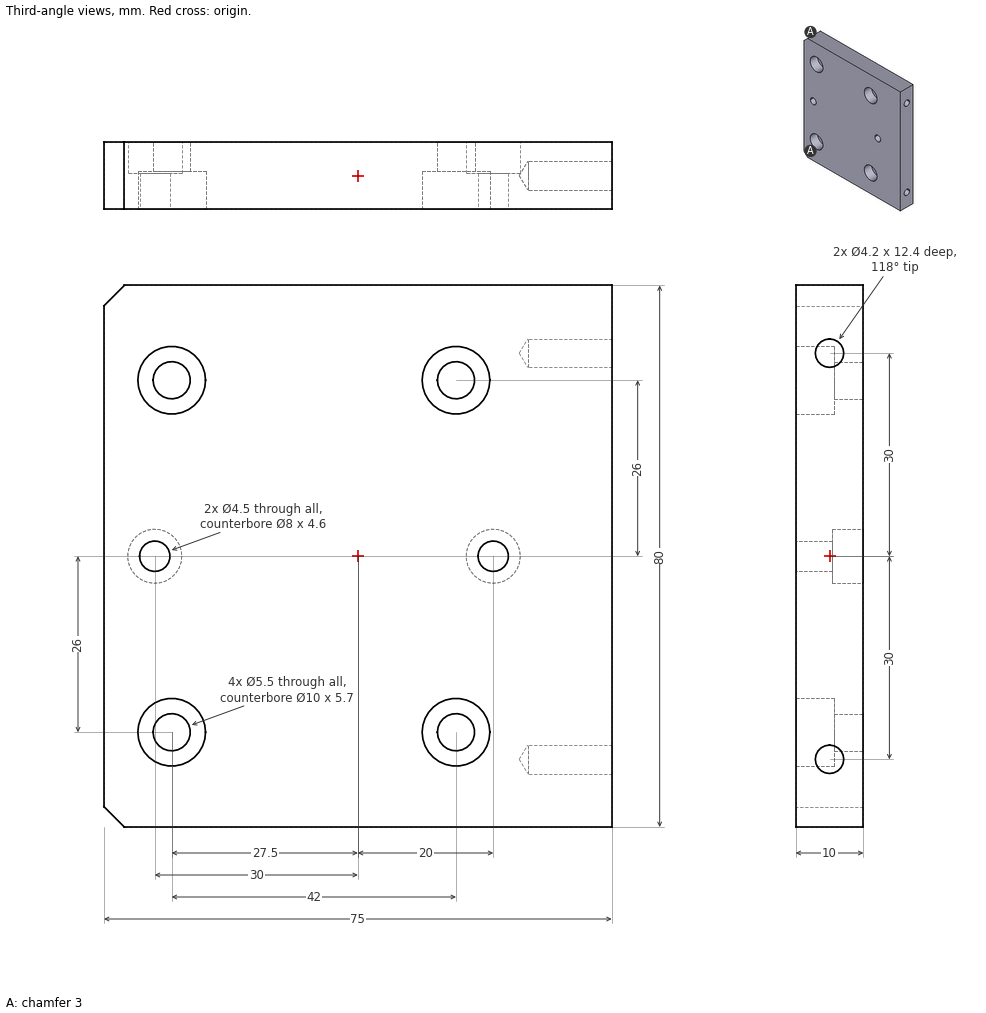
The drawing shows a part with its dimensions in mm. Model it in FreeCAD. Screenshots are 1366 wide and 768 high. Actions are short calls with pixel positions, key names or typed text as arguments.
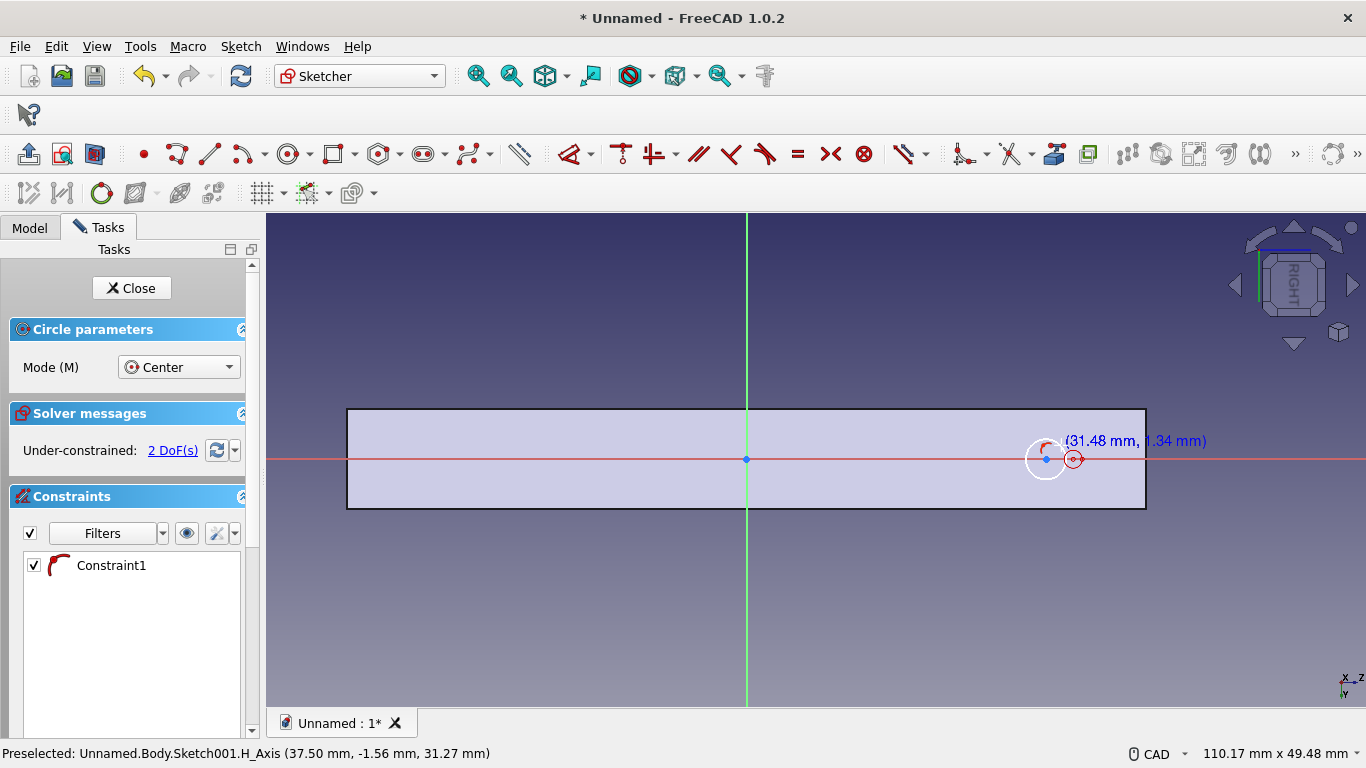
click(447, 459)
click(462, 445)
key(Escape)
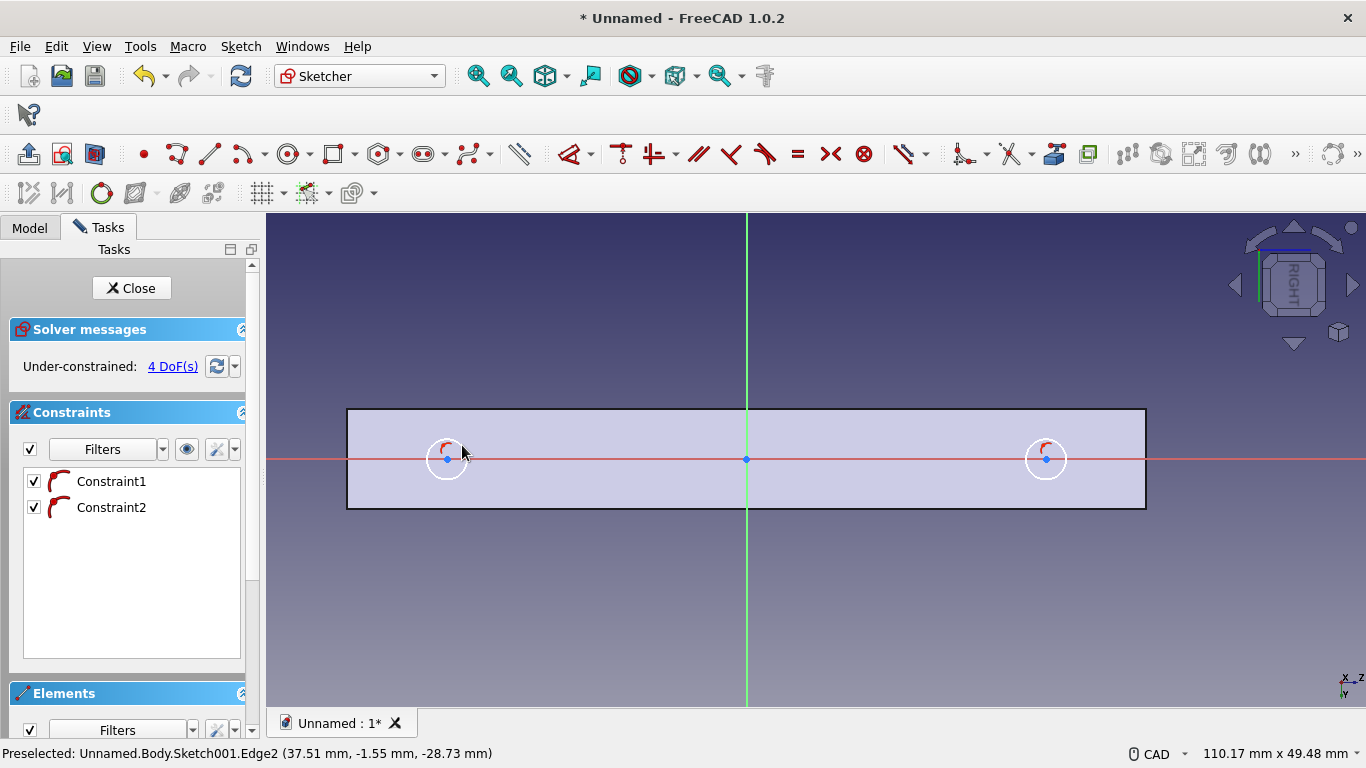
click(1060, 445)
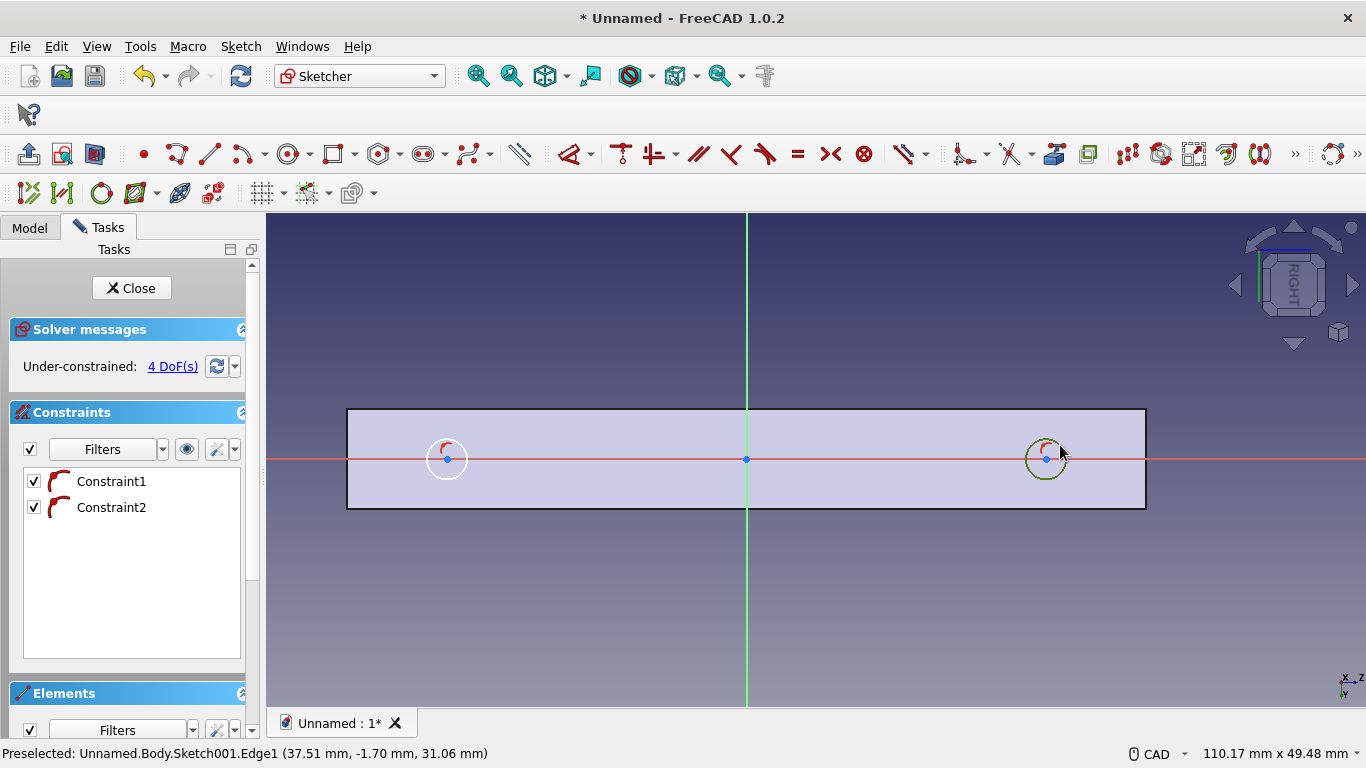
click(461, 445)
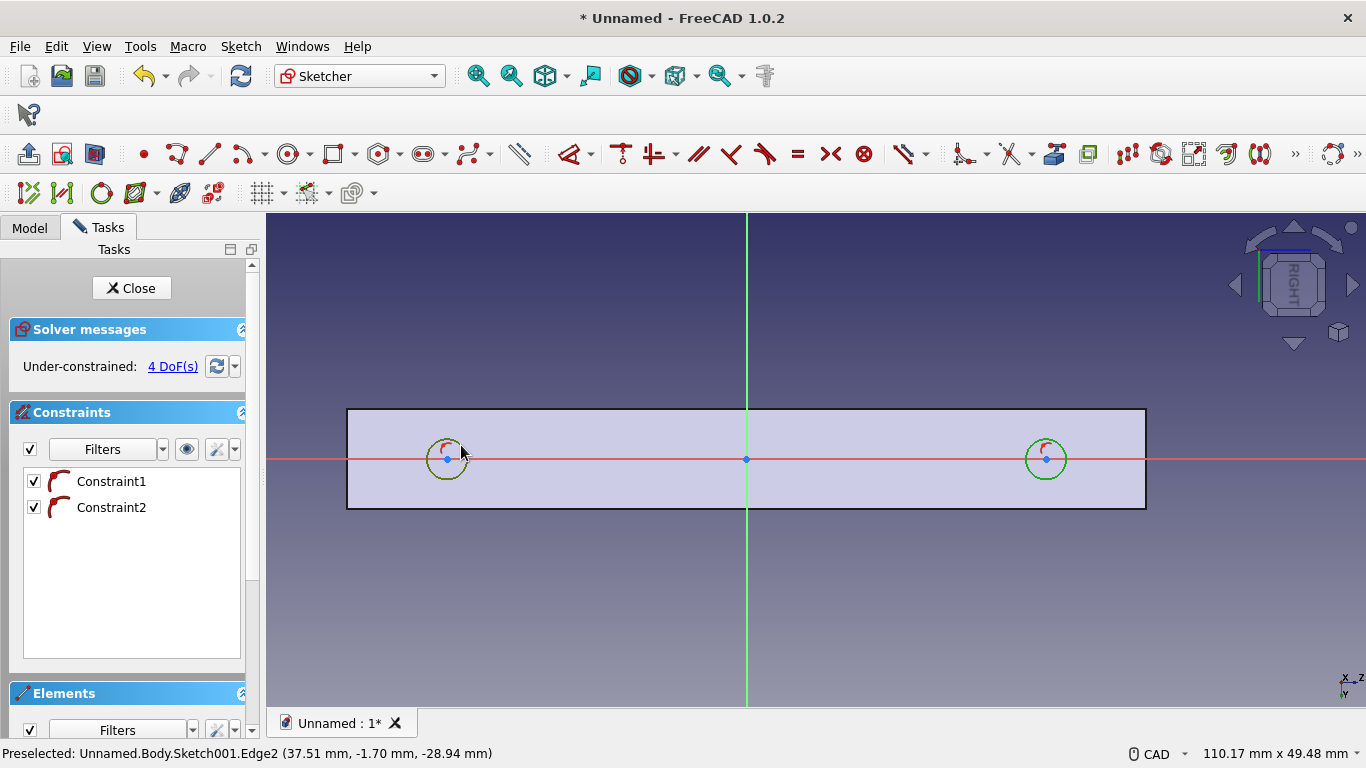
click(798, 154)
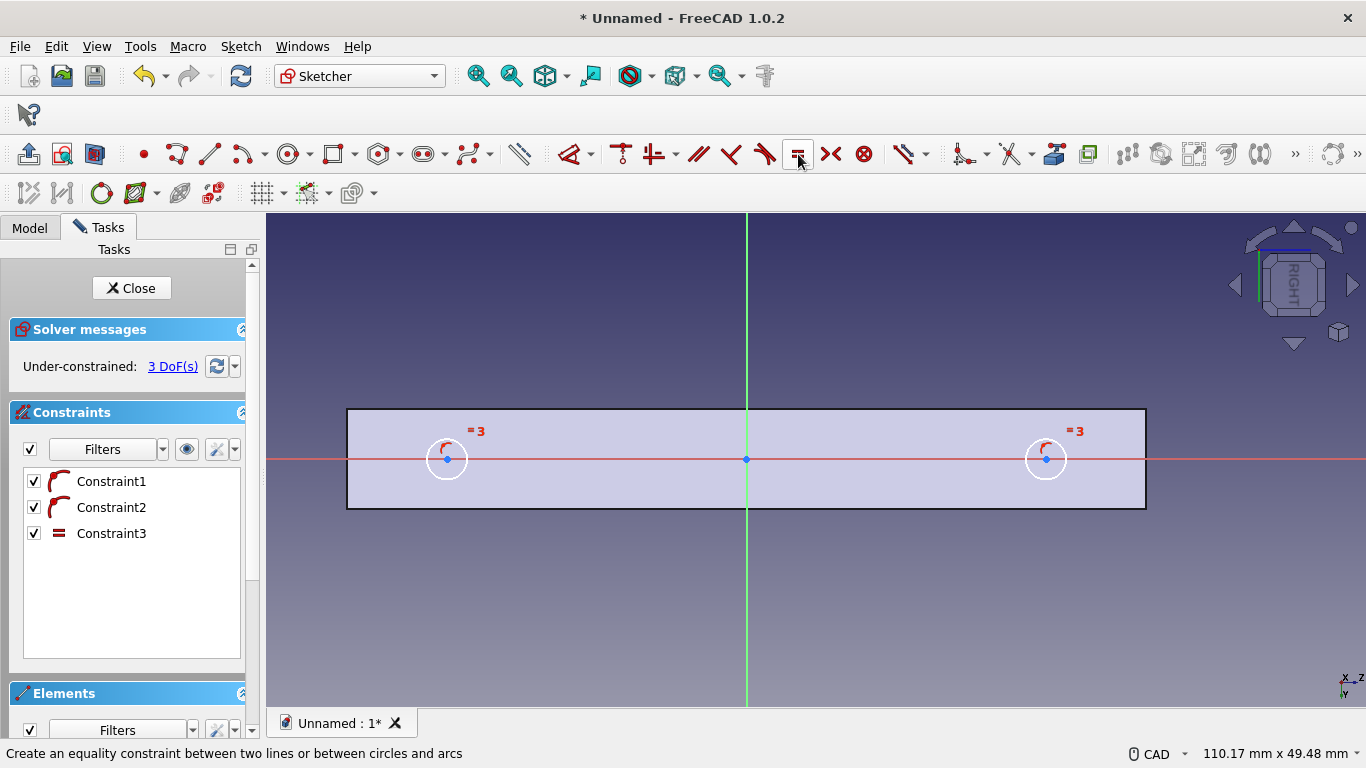
click(568, 154)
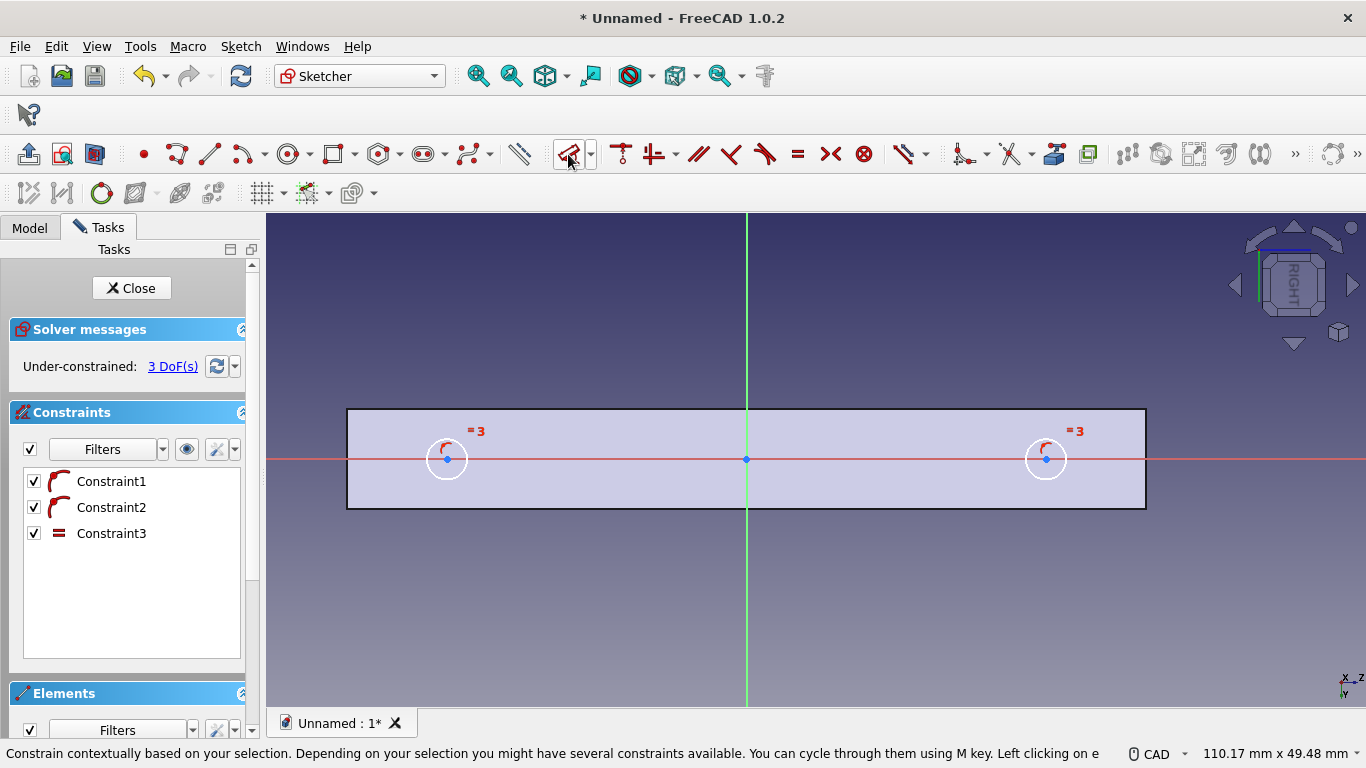
click(1060, 445)
click(1082, 422)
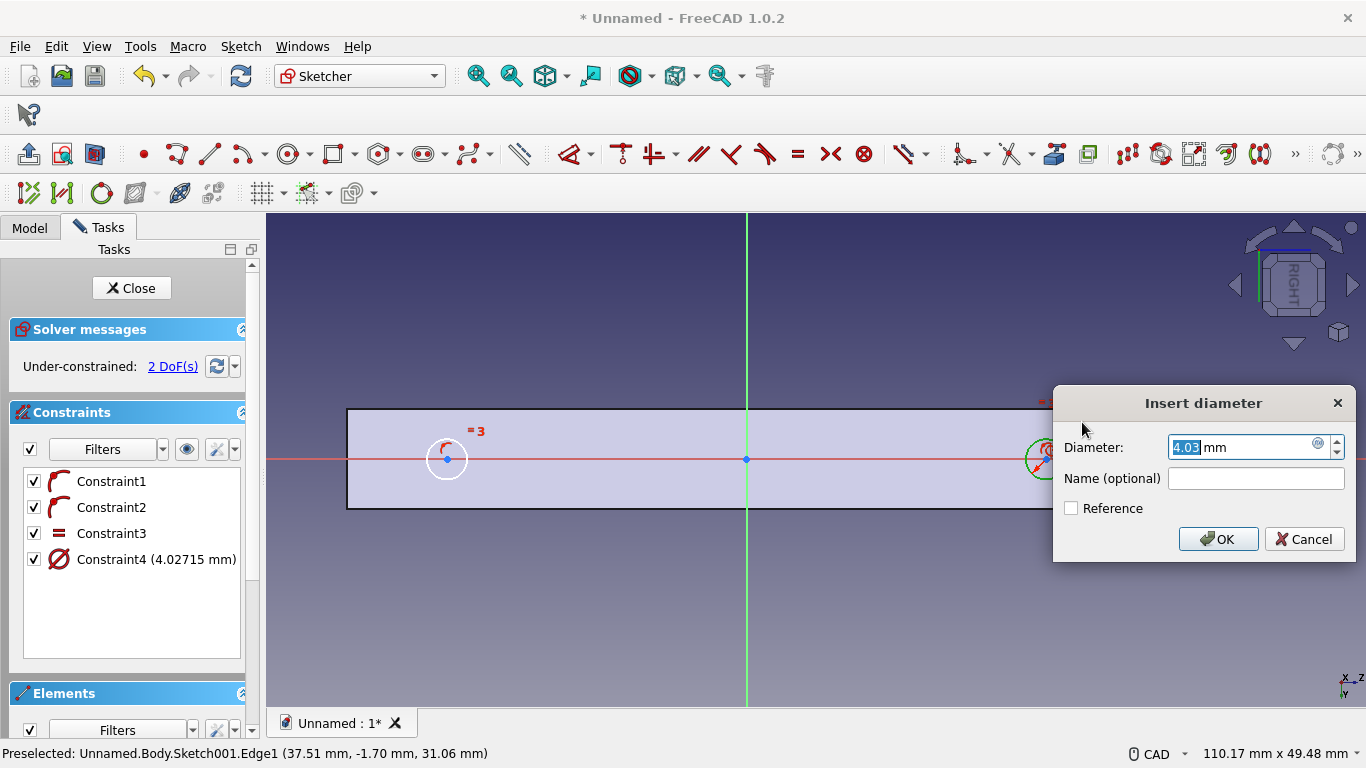
text(4.2)
key(Return)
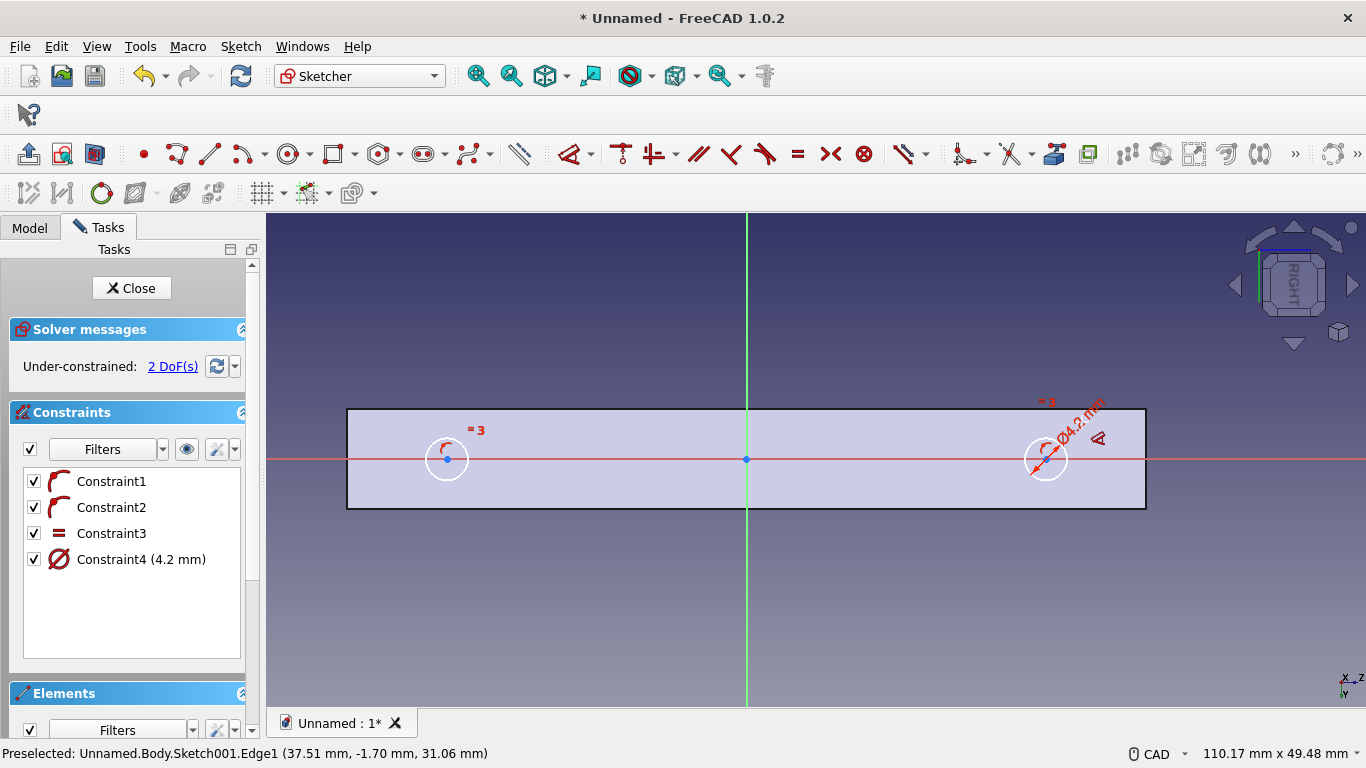
click(1046, 459)
click(896, 493)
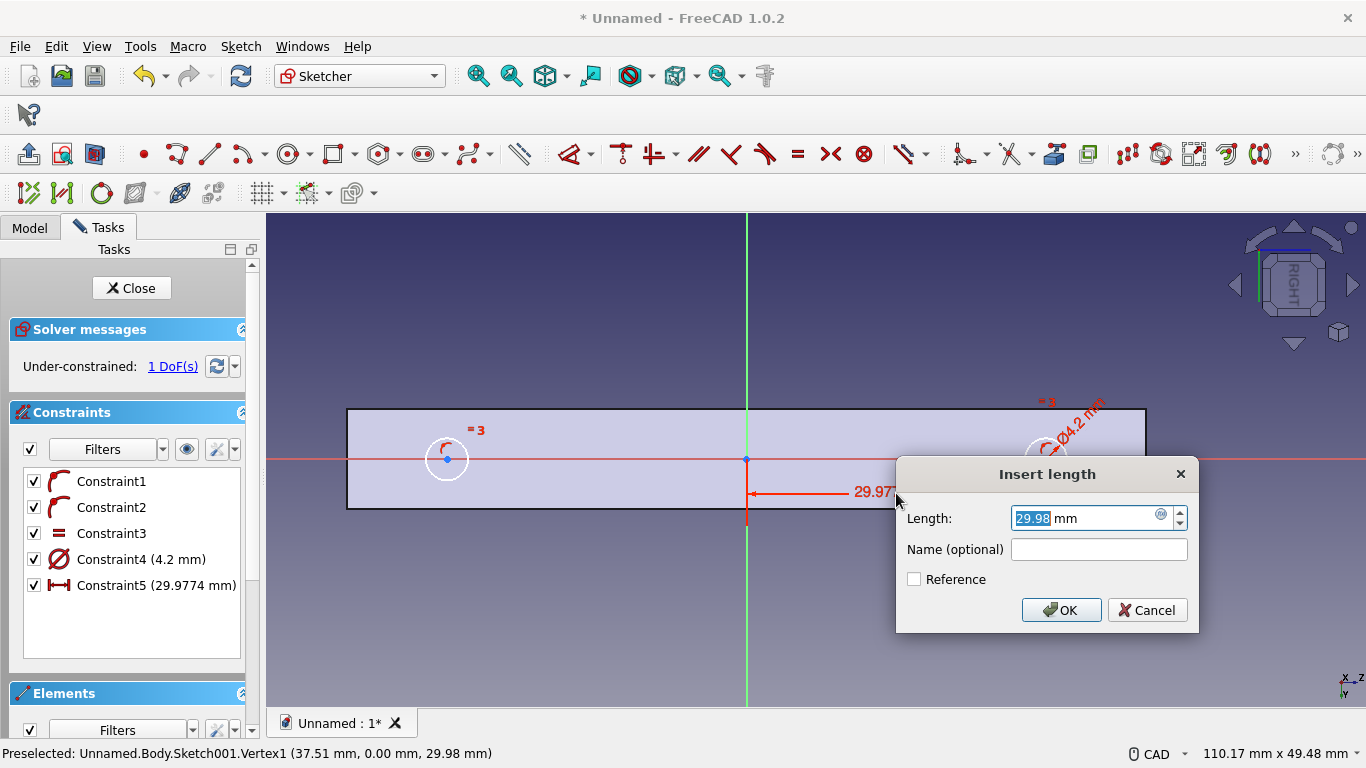
text(30)
key(Return)